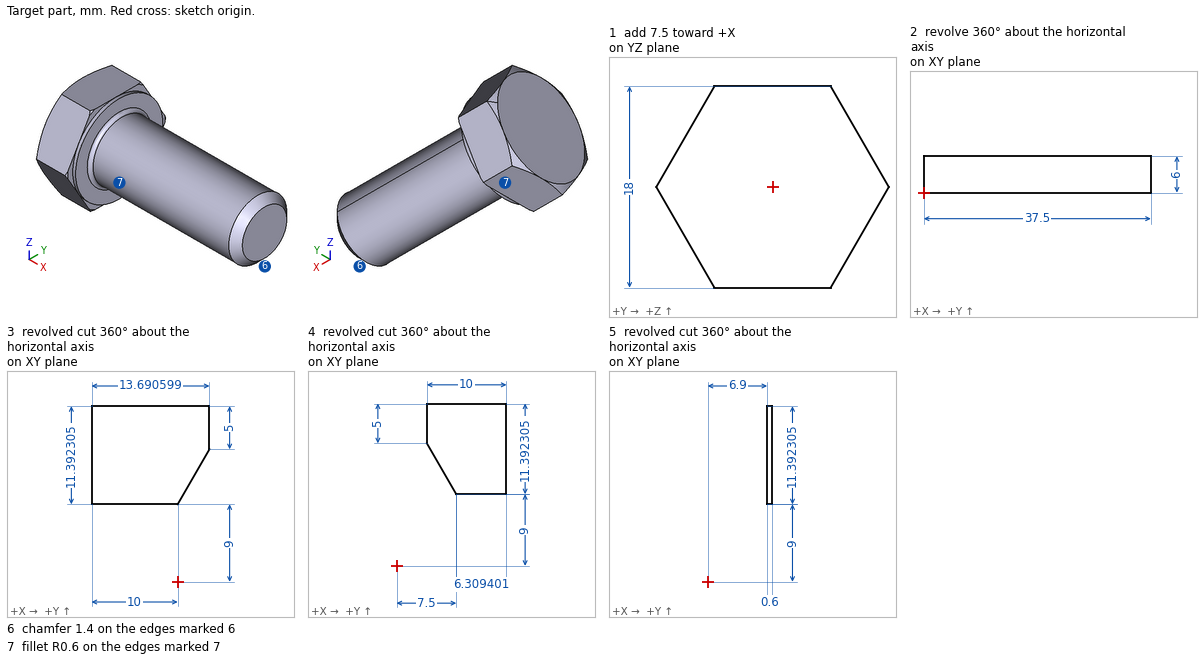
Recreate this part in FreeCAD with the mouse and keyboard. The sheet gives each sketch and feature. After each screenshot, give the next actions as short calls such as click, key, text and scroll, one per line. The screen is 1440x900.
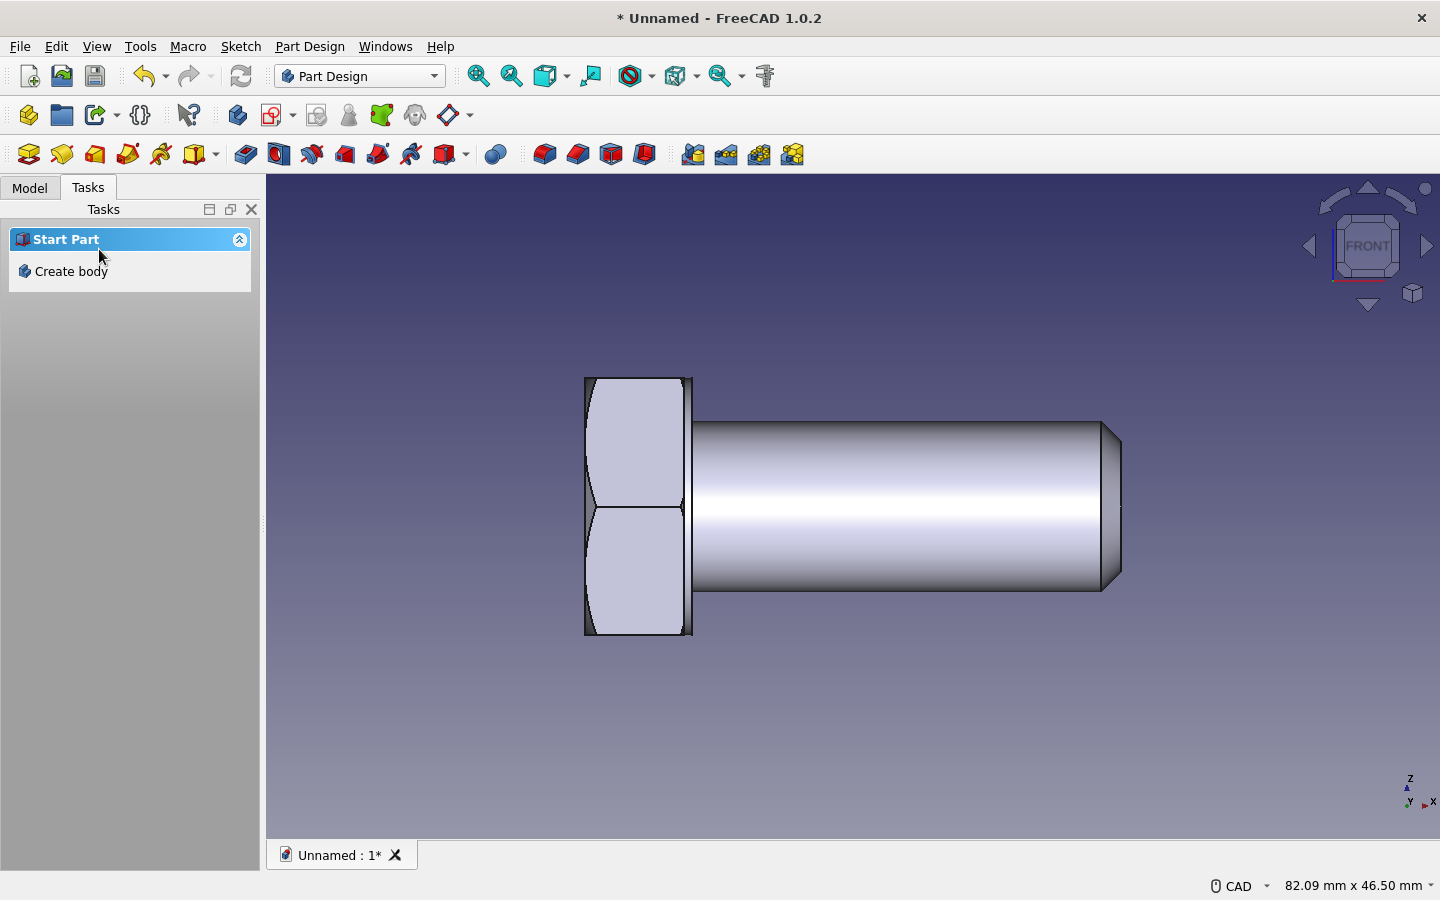
key(3)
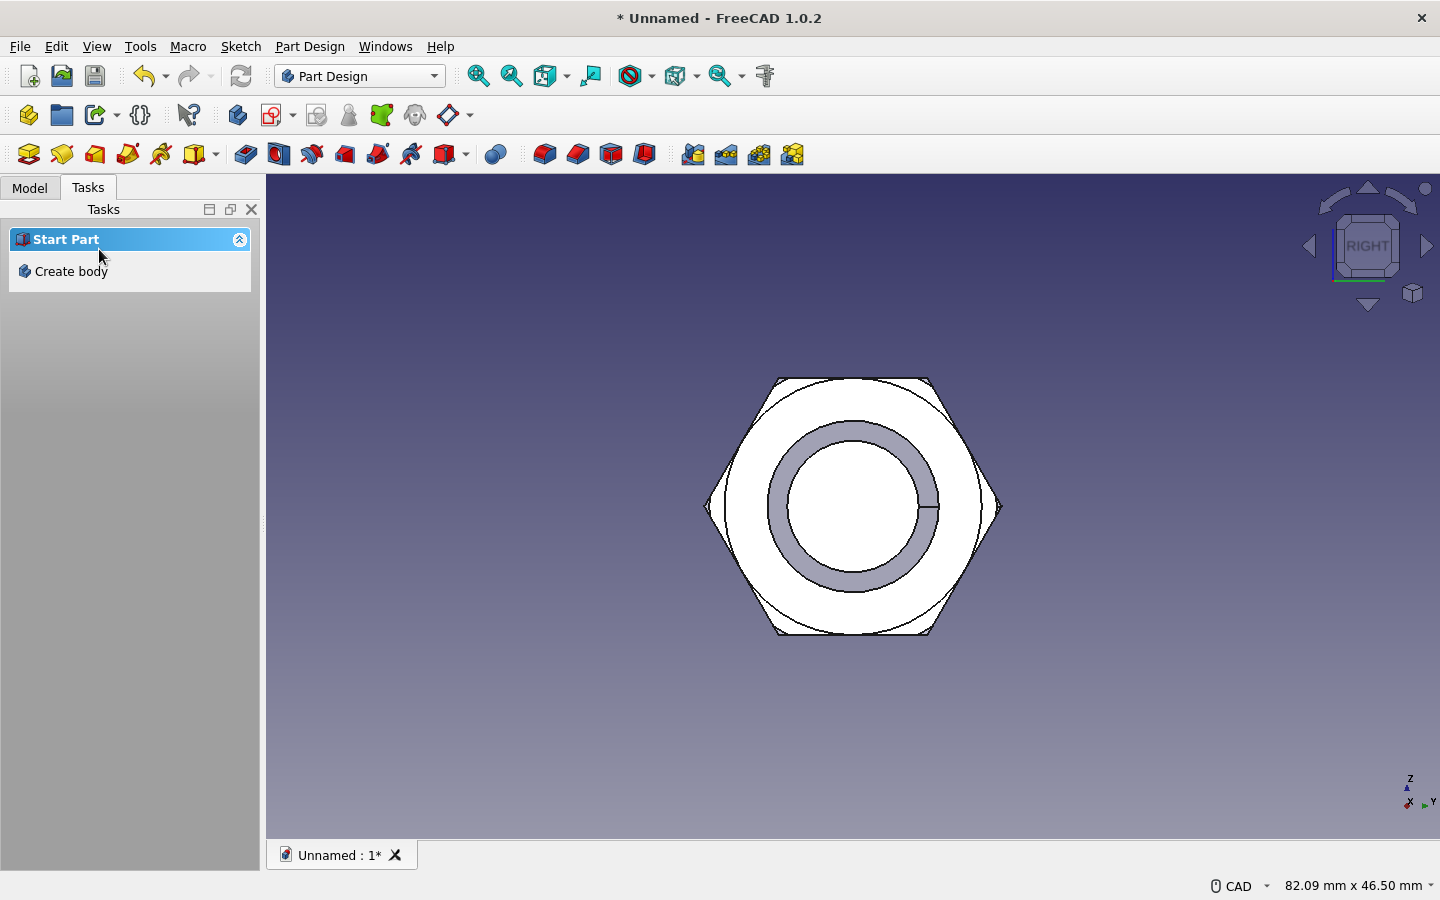
key(v)
key(f)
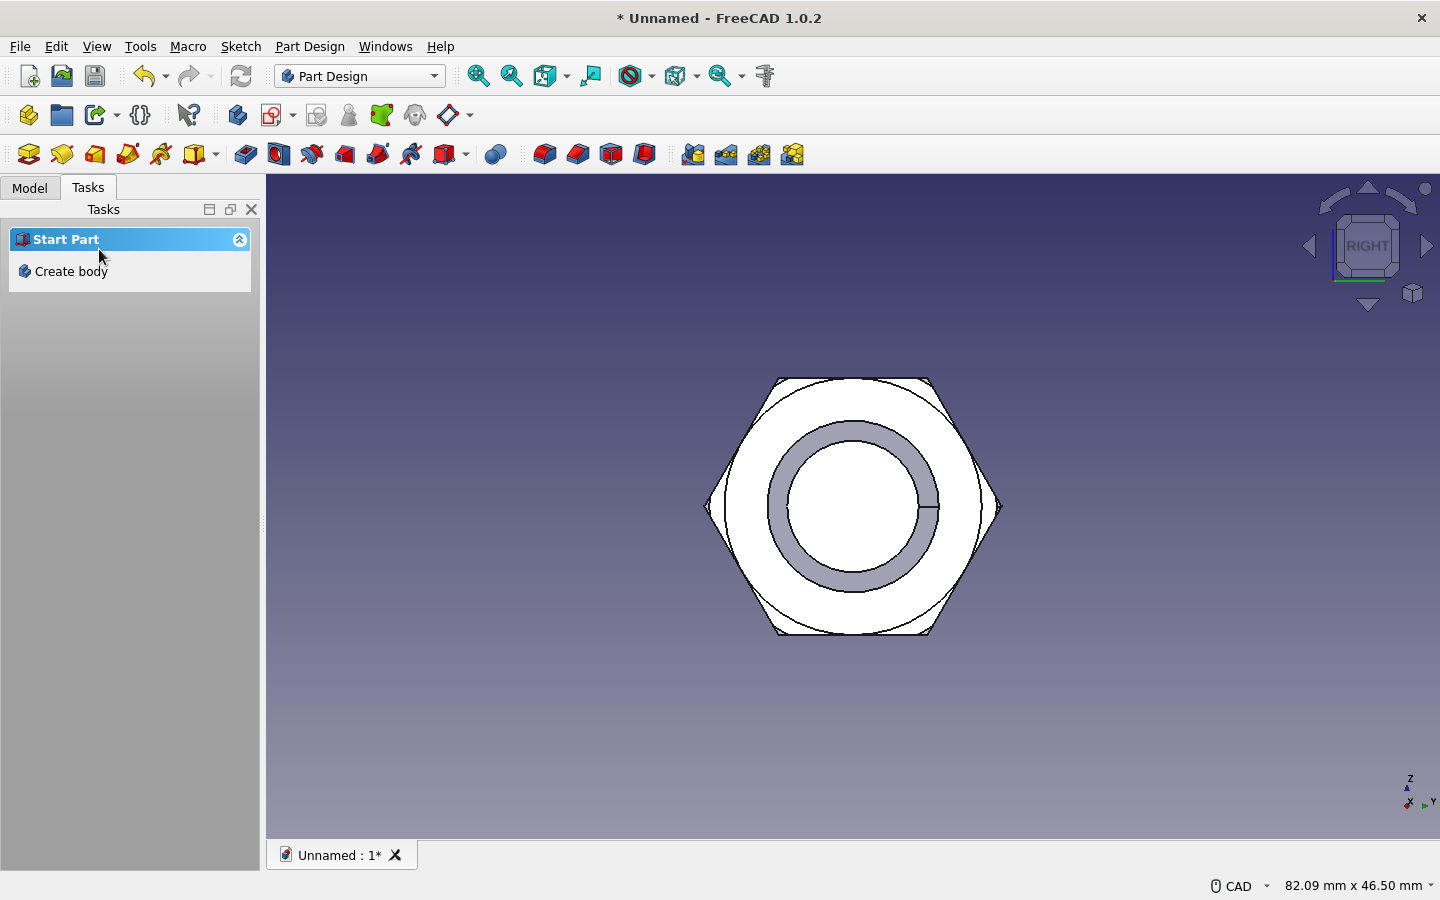
key(5)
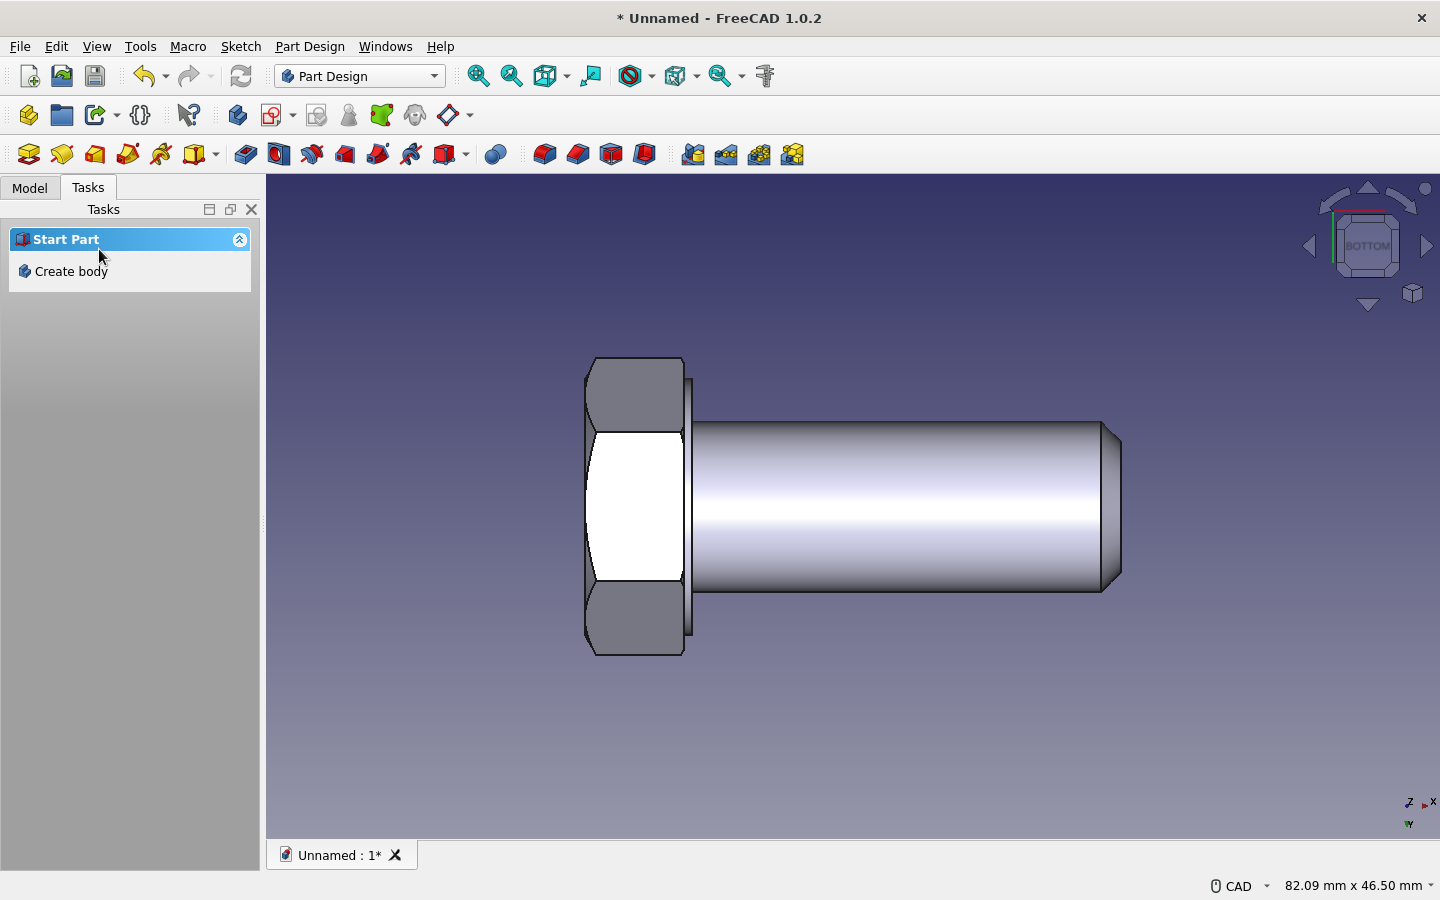
key(4)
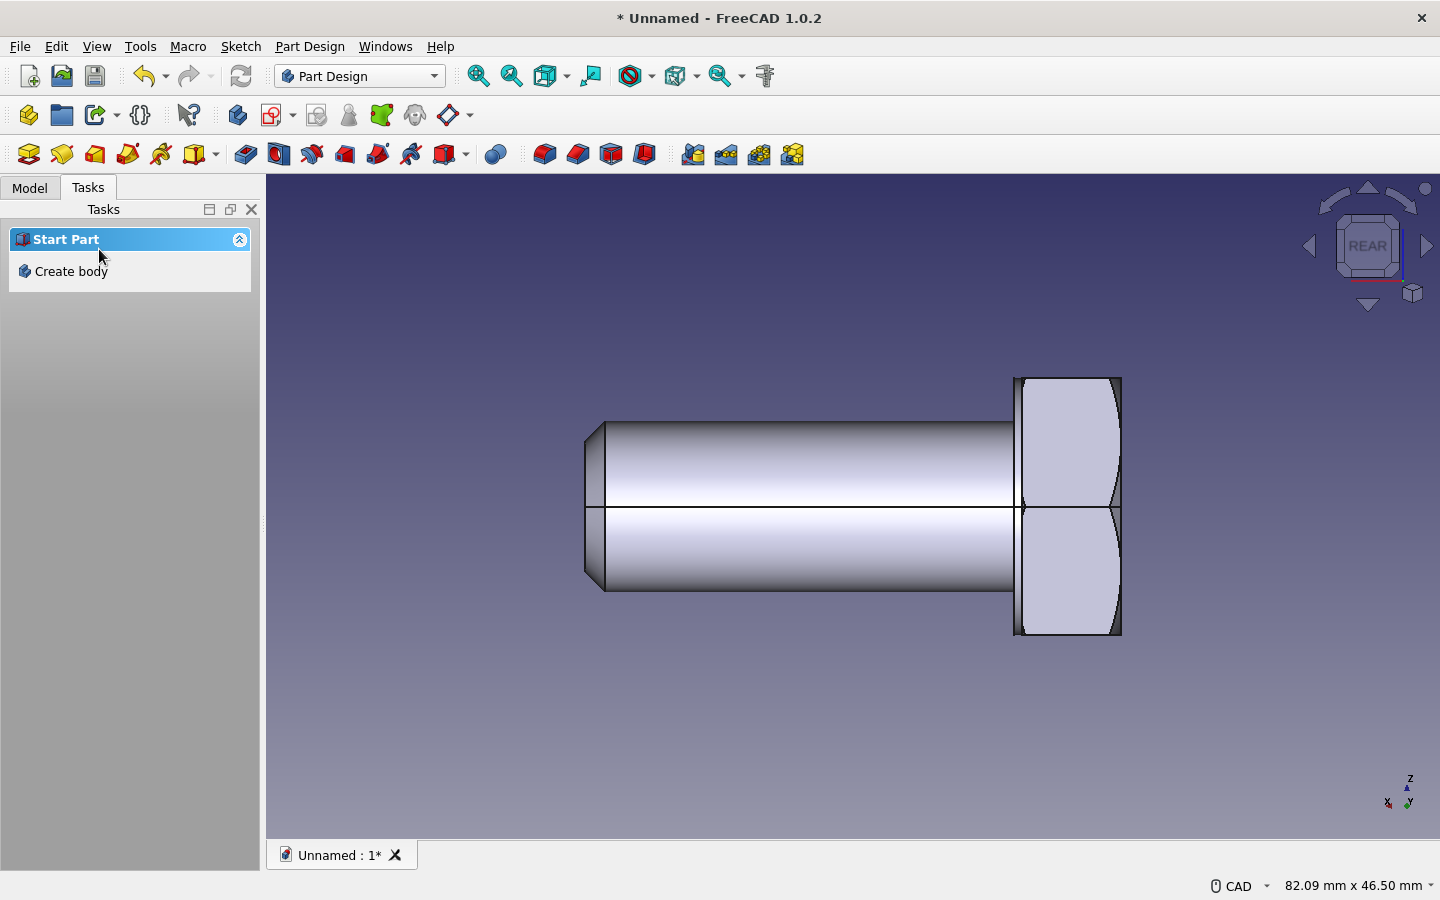
key(6)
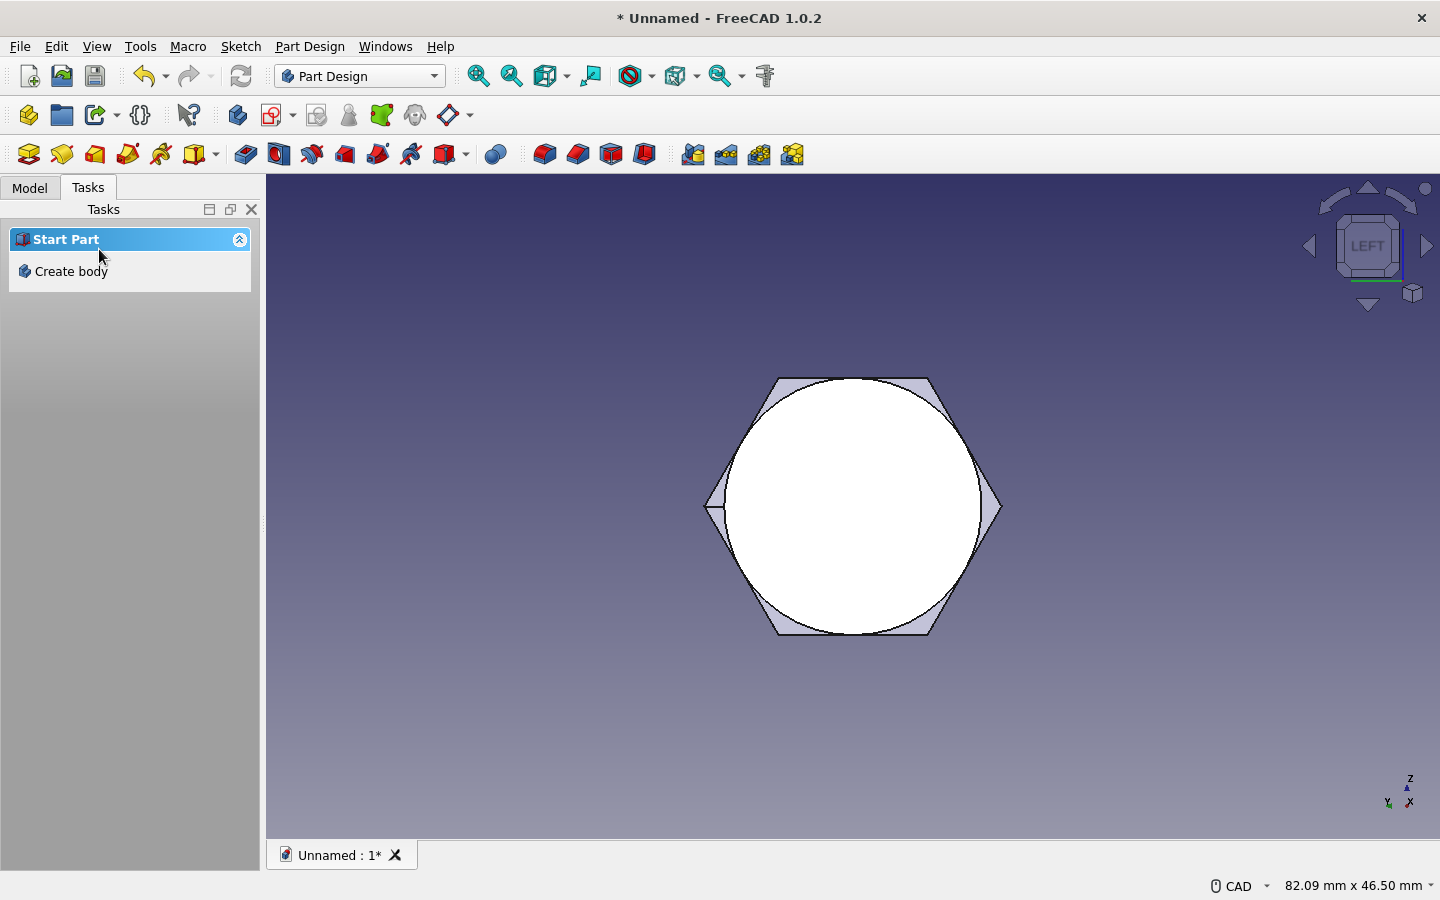
key(v)
key(f)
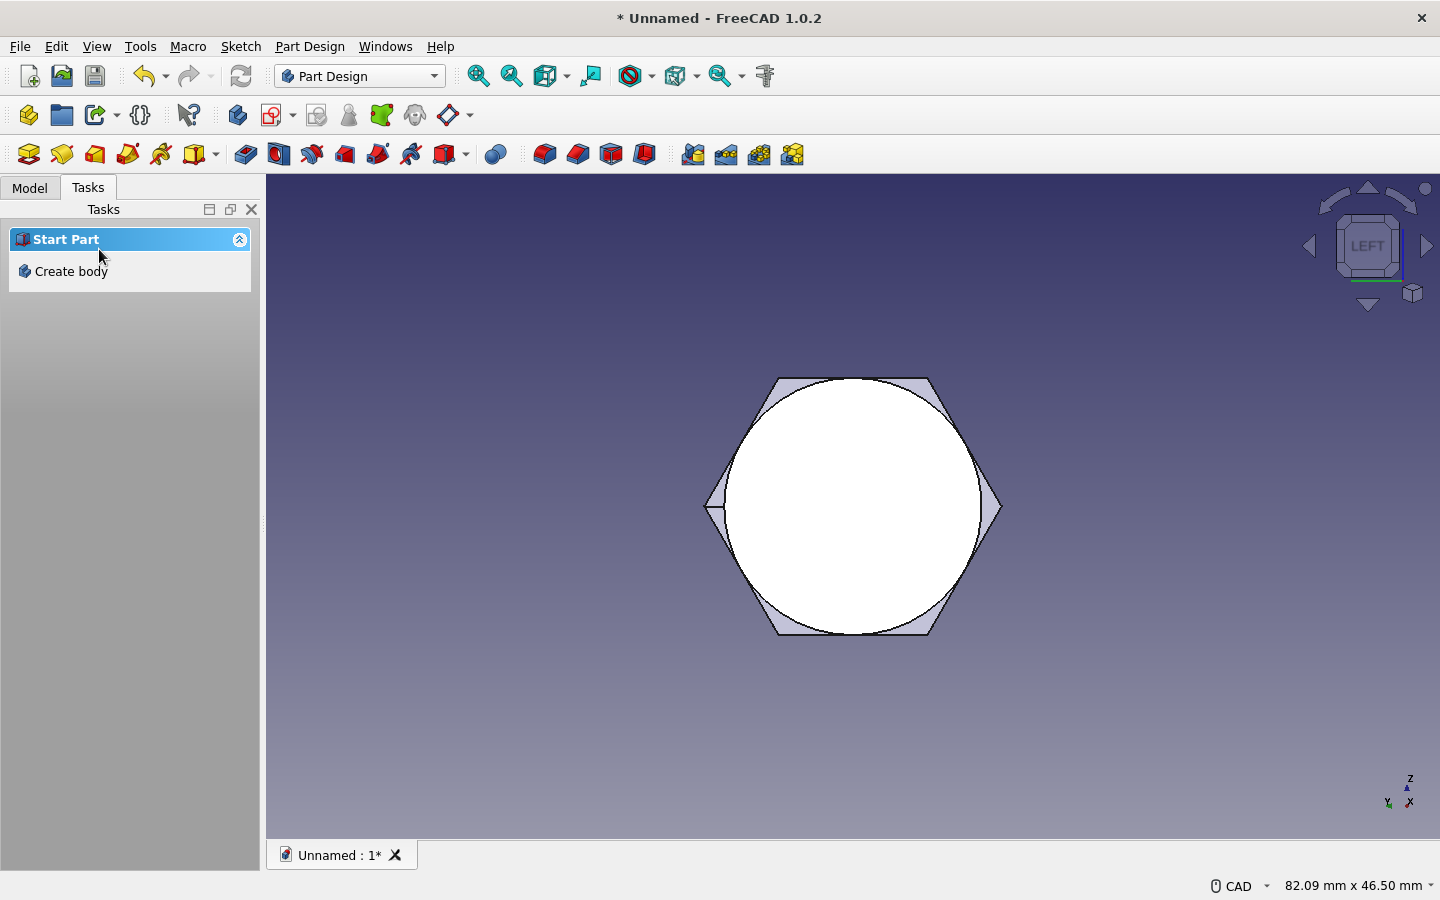
key(v)
key(3)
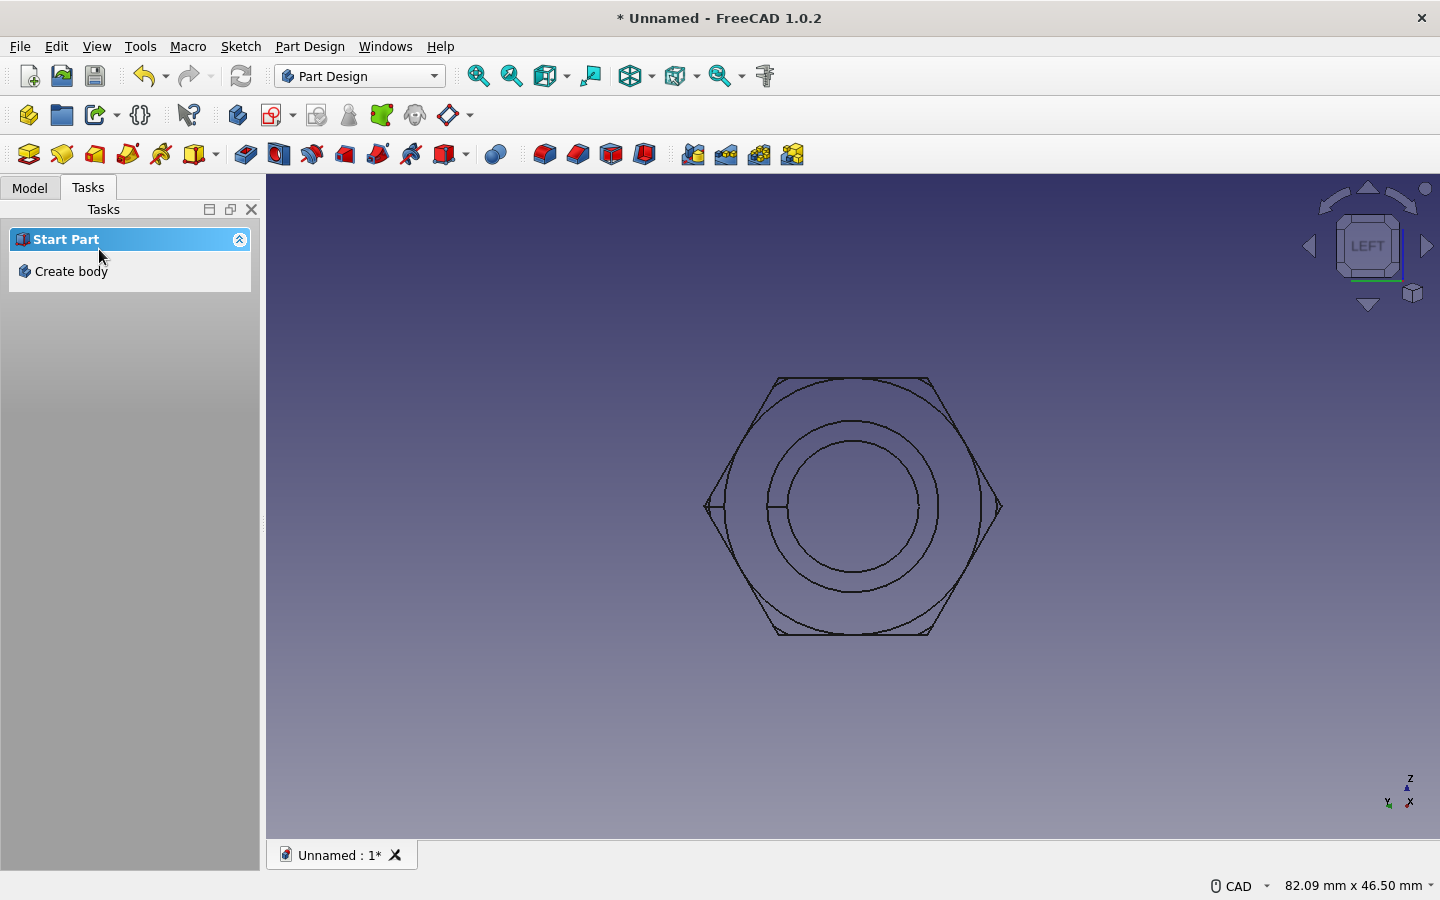
key(0)